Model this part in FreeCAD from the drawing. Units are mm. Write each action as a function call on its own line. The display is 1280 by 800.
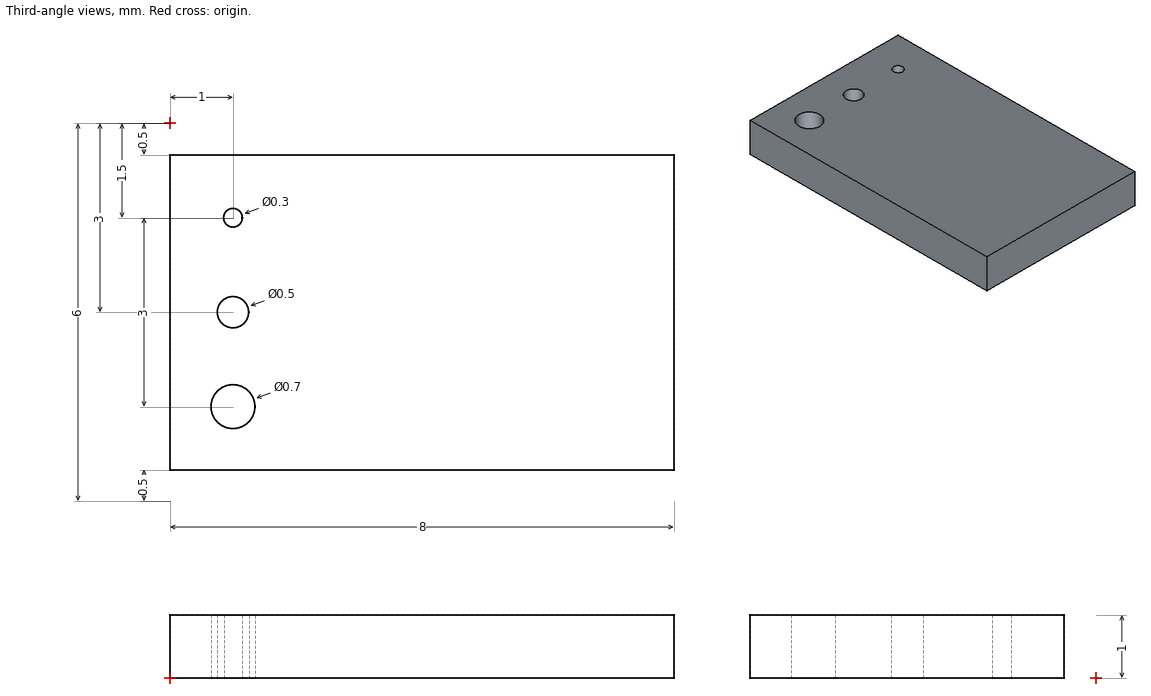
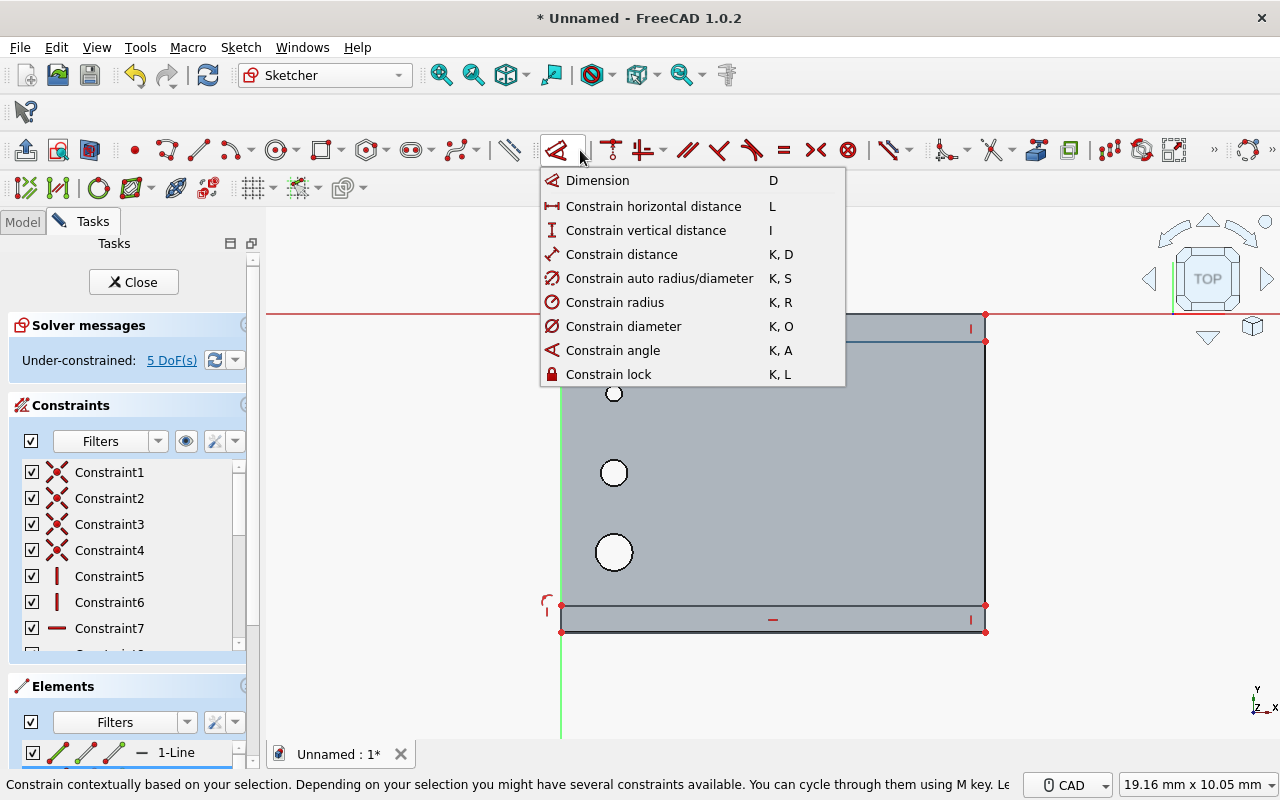
click(693, 206)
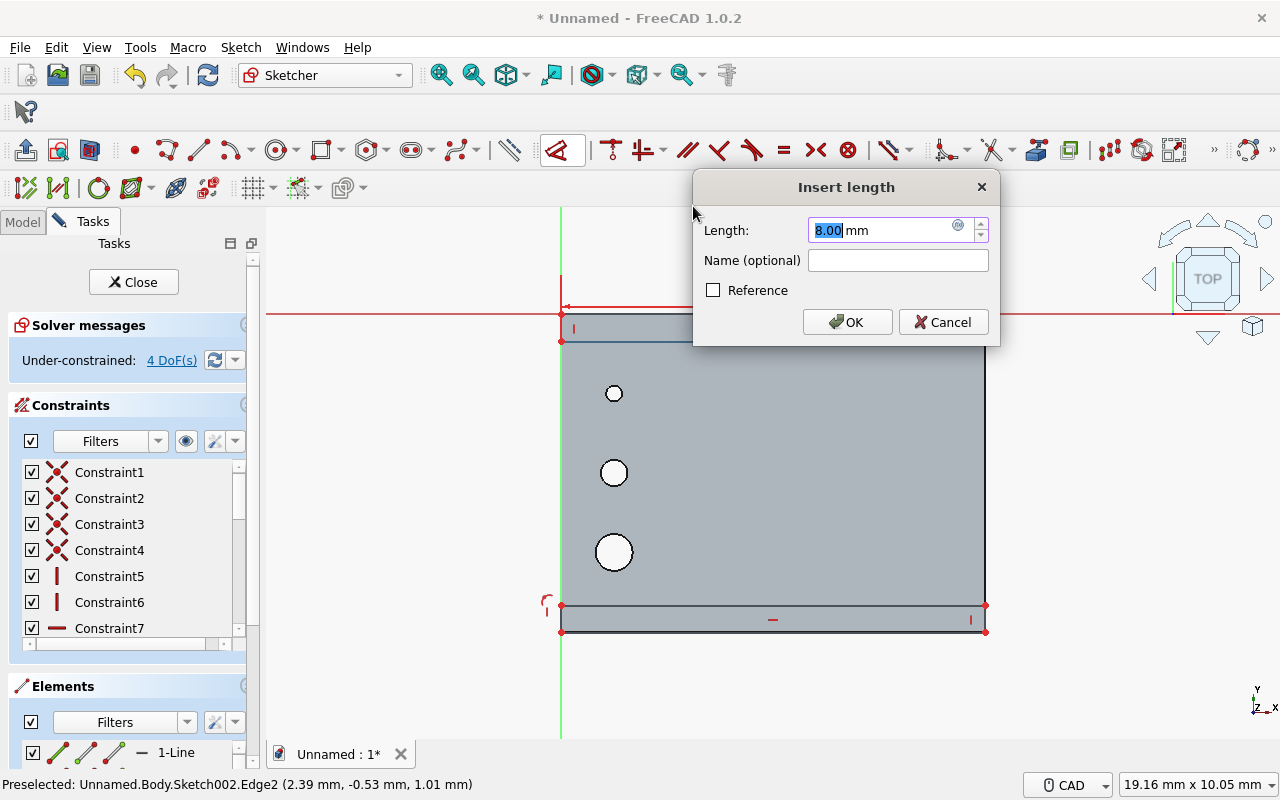
text(8)
key(Return)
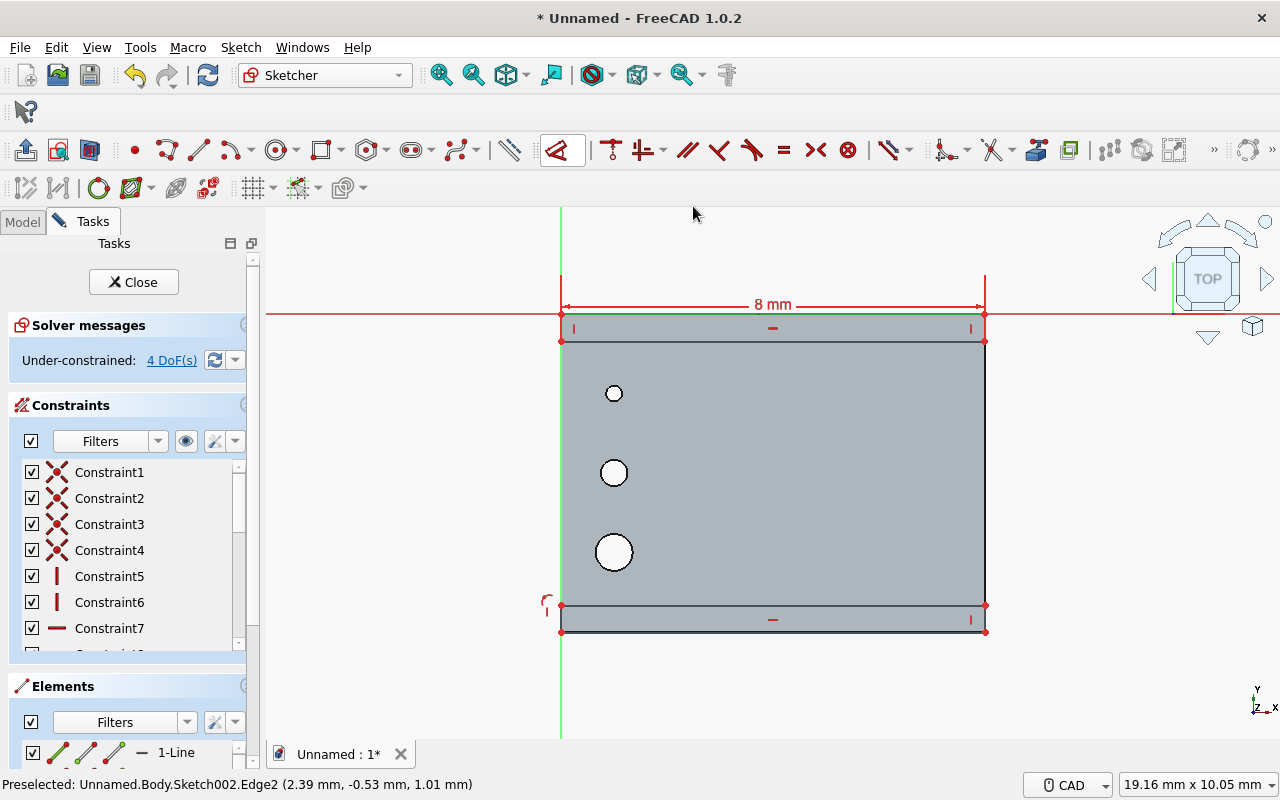
click(688, 633)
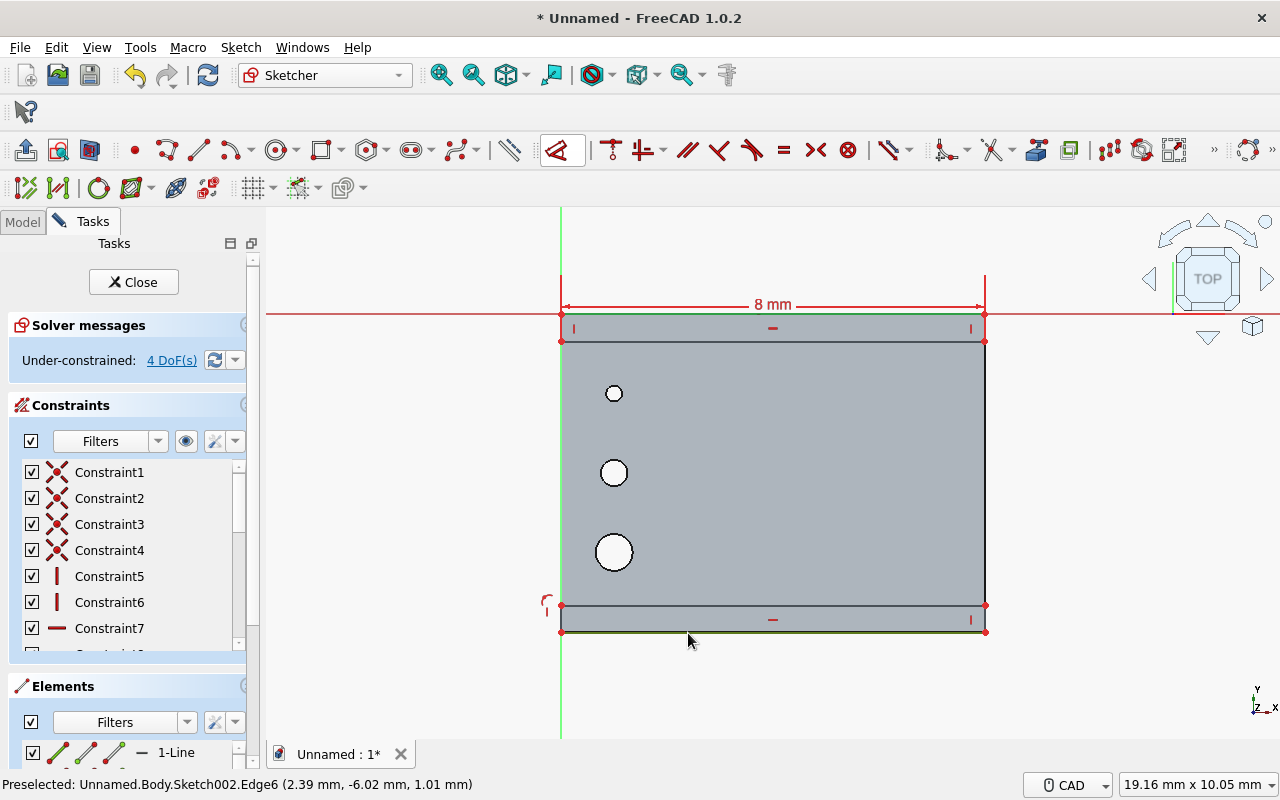
key(l)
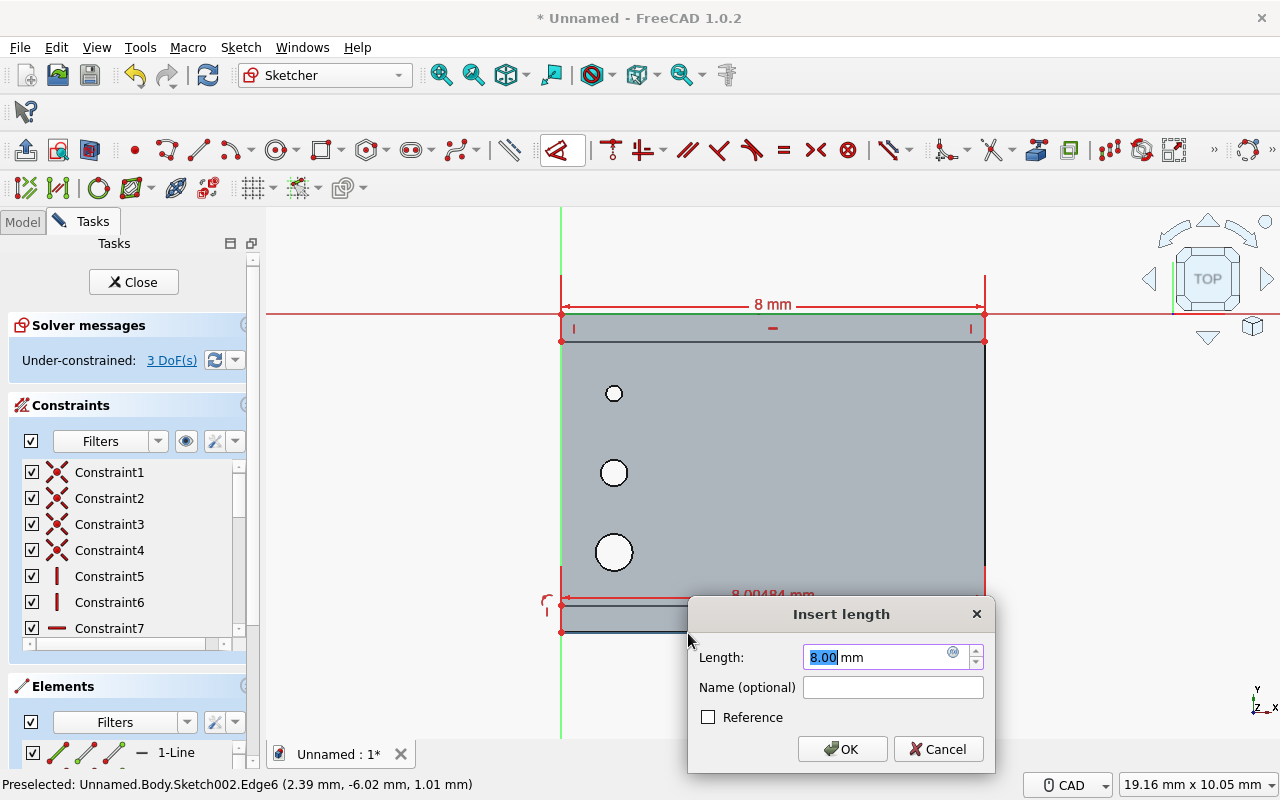
text(8)
key(Return)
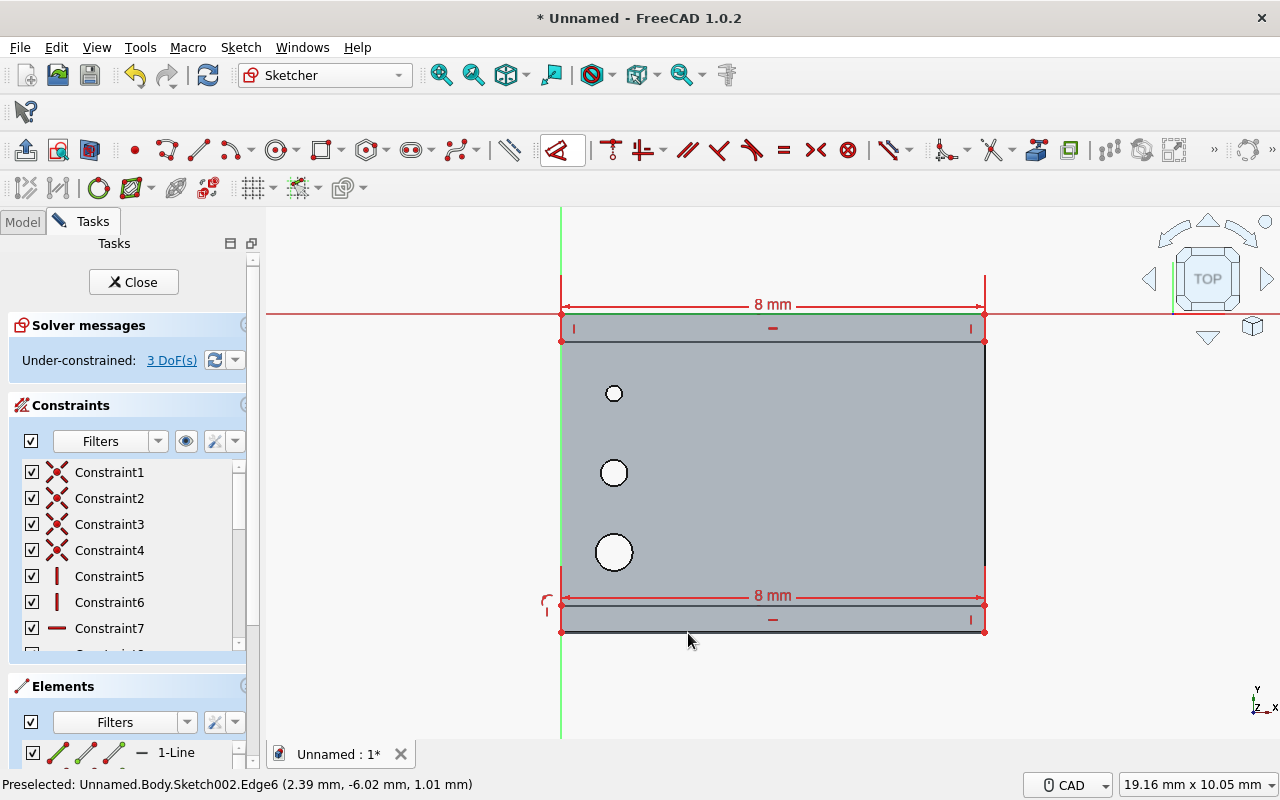
click(561, 633)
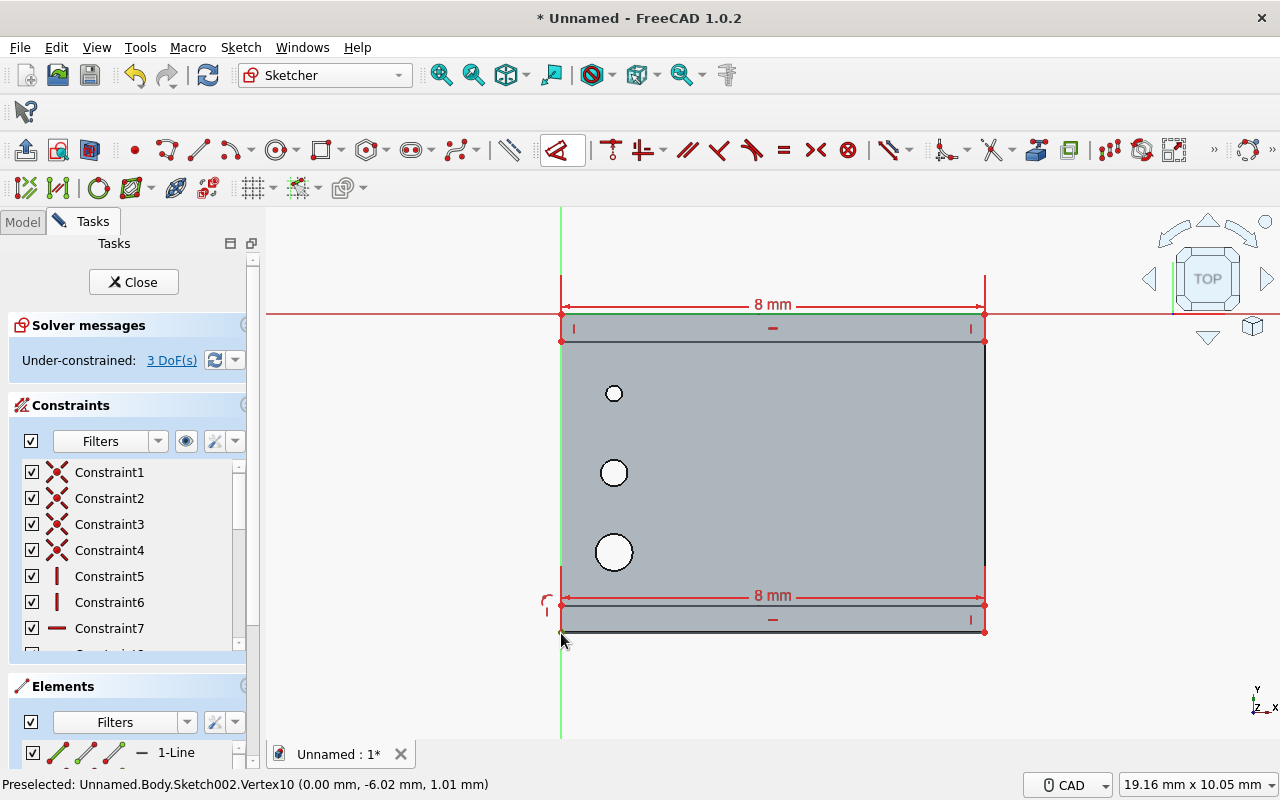
key(i)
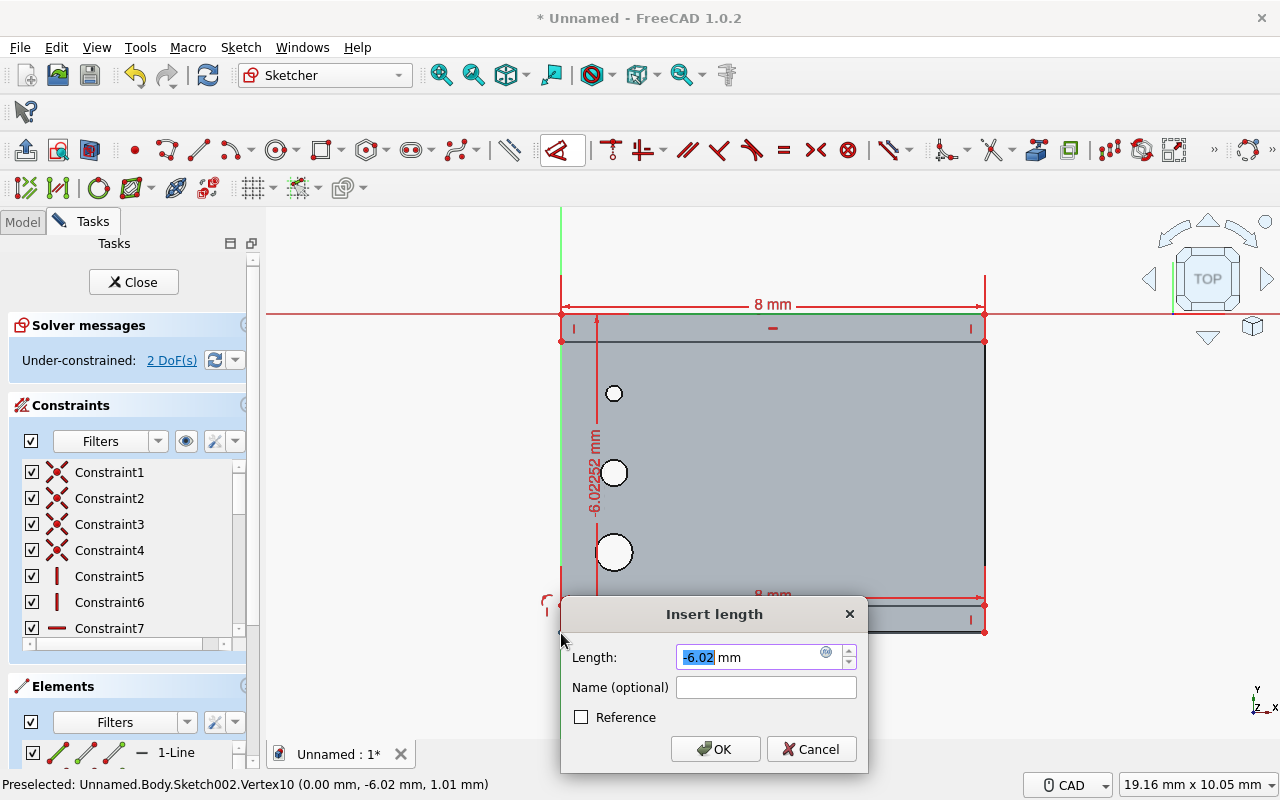
text(-6)
key(Return)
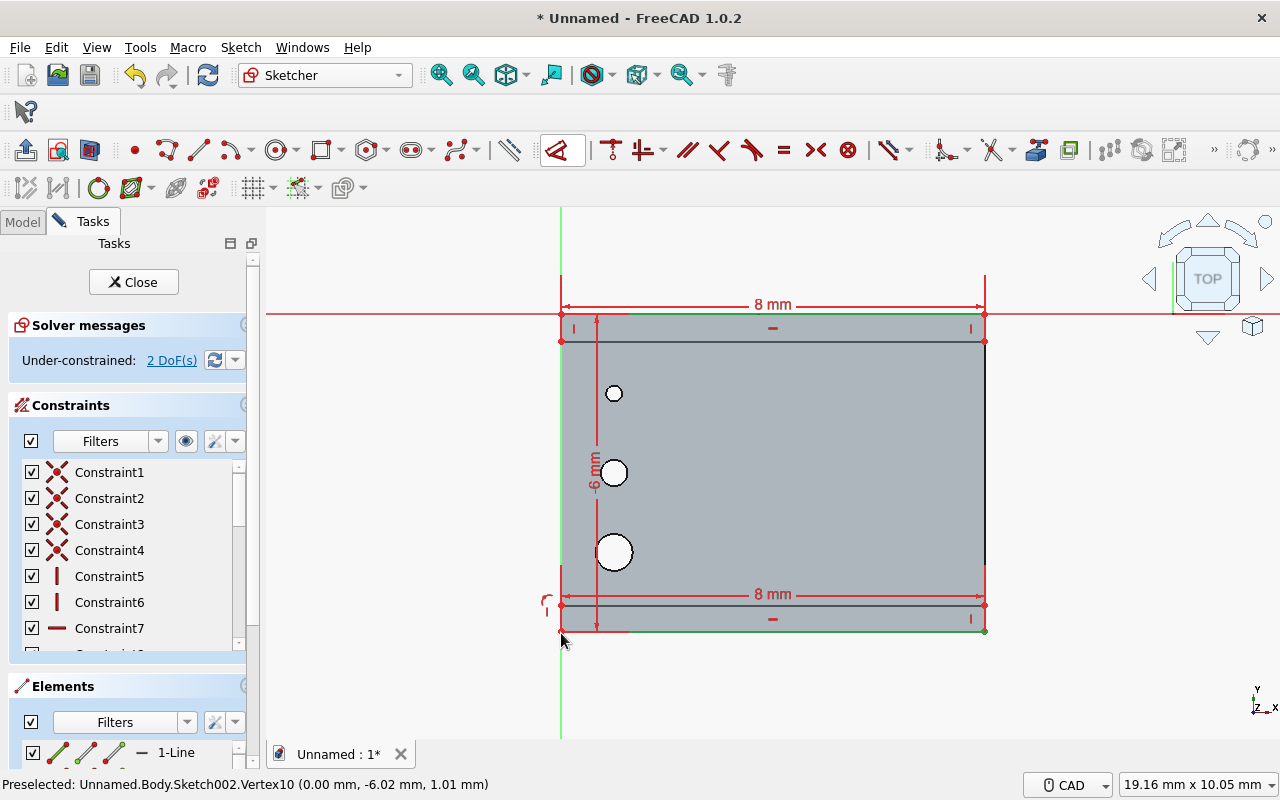
scroll(561, 325, up, 3)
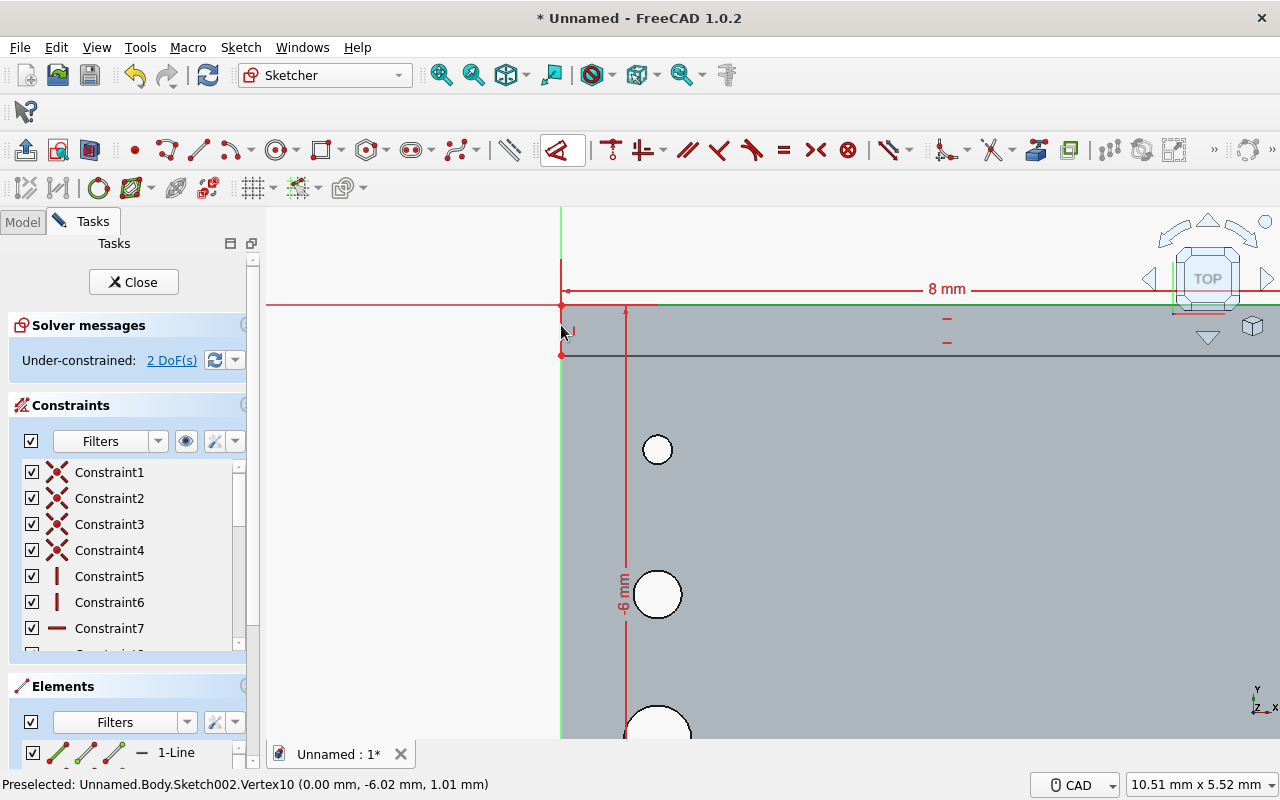
click(561, 325)